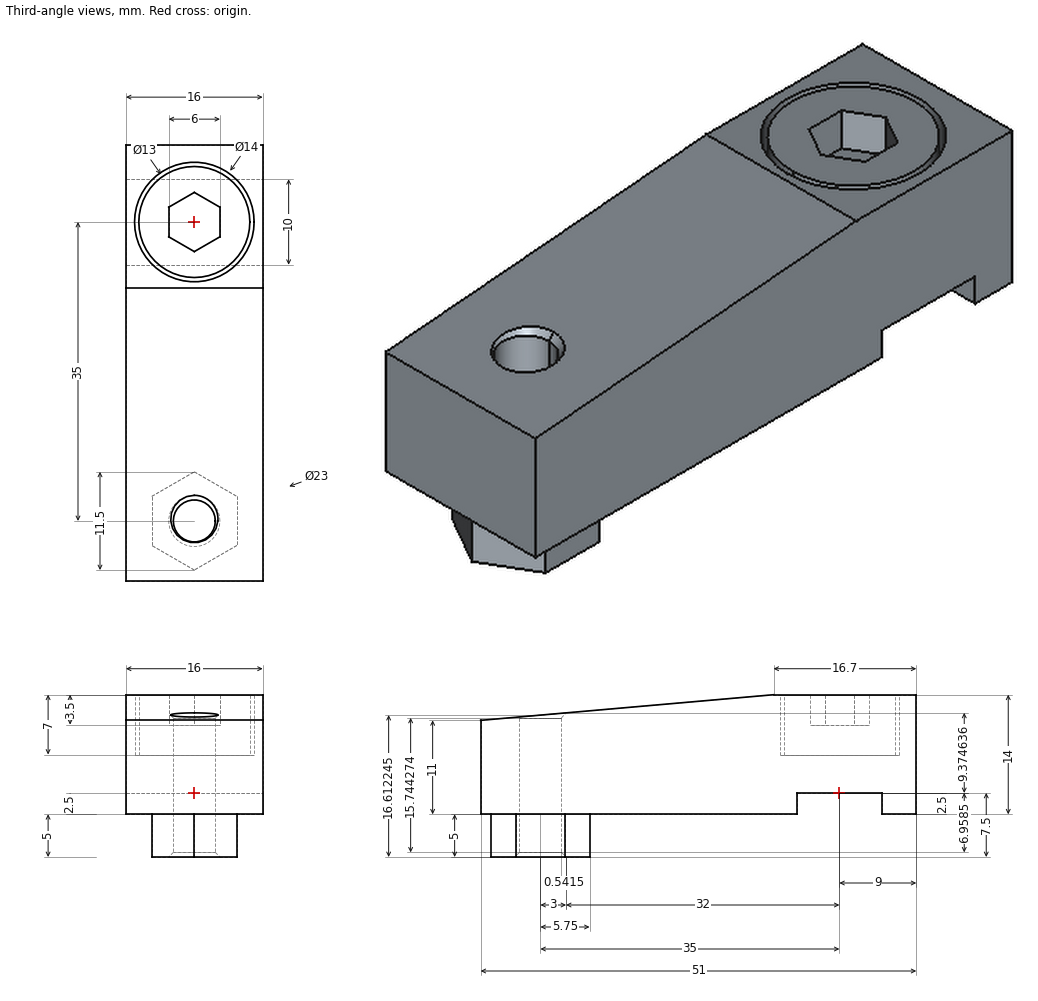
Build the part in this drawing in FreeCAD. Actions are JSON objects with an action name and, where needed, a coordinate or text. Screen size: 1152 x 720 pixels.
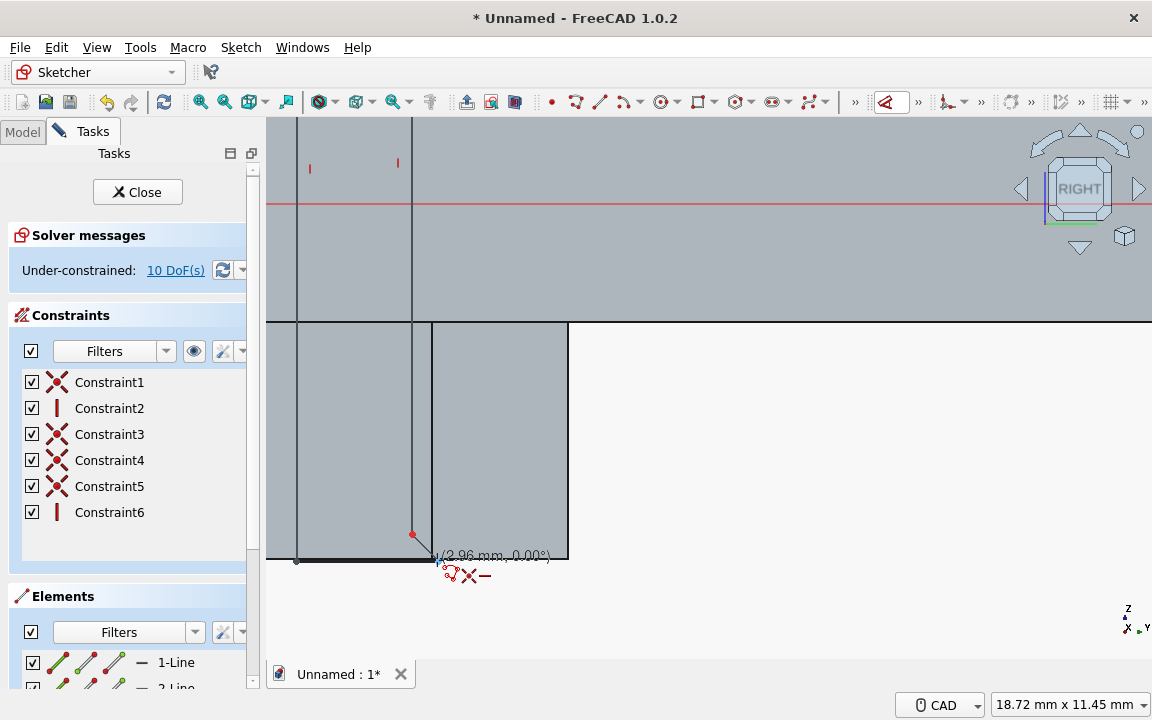
{"action": "left_click", "coordinate": [439, 561]}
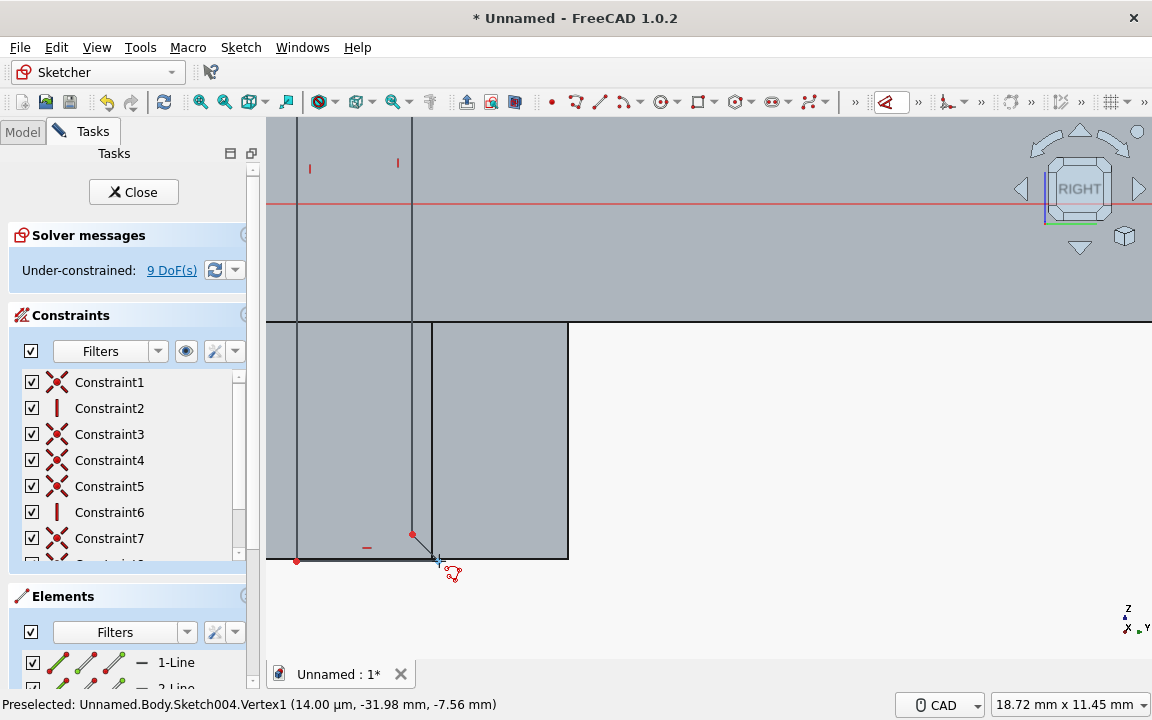
{"action": "left_click", "coordinate": [600, 102]}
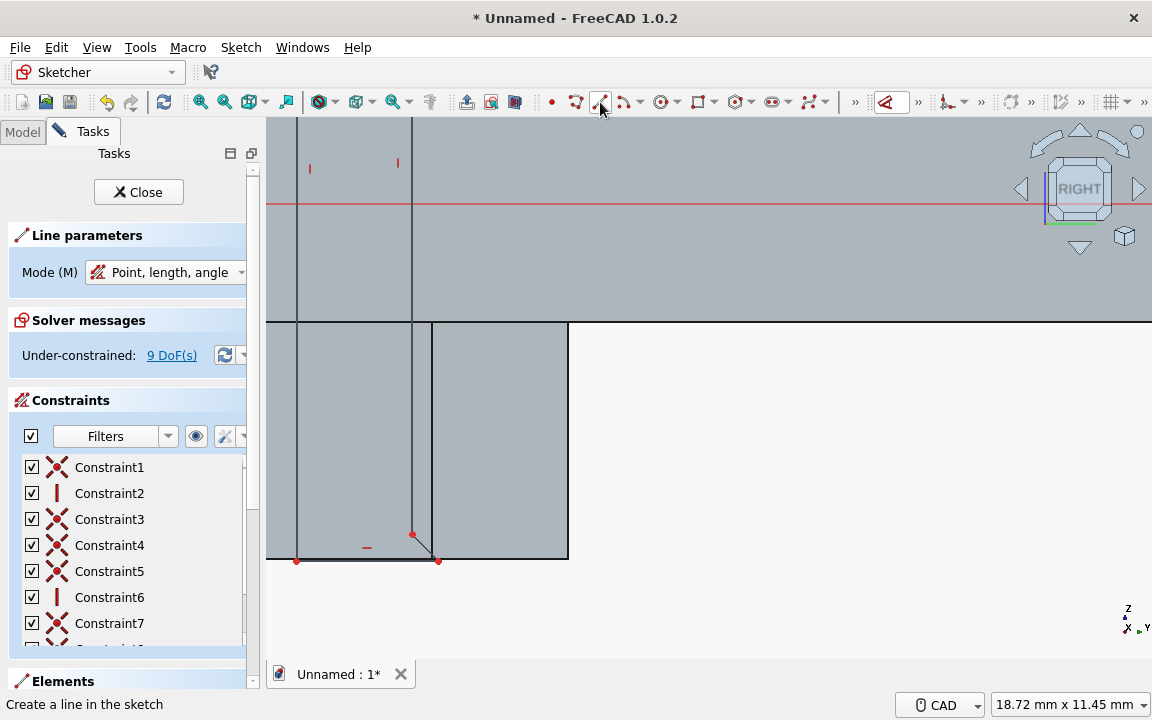
{"action": "scroll", "coordinate": [432, 555], "scroll_direction": "down", "scroll_amount": 6}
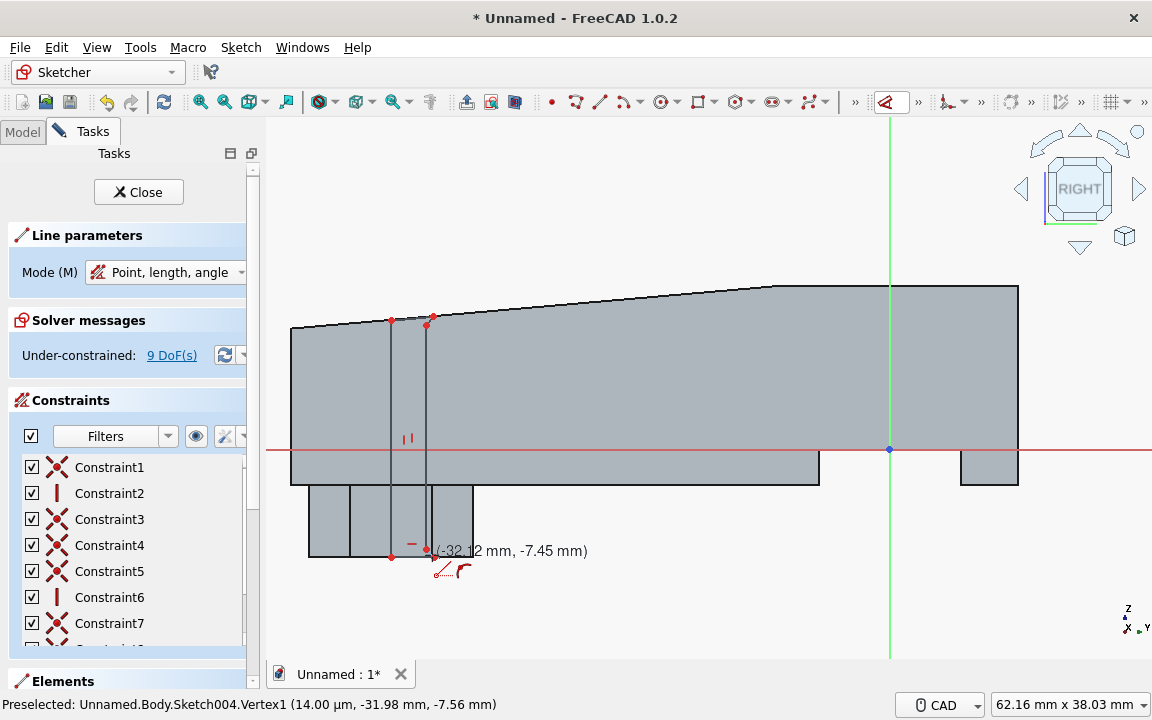
{"action": "left_click", "coordinate": [391, 292]}
{"action": "left_click", "coordinate": [391, 220]}
{"action": "key", "text": "Escape"}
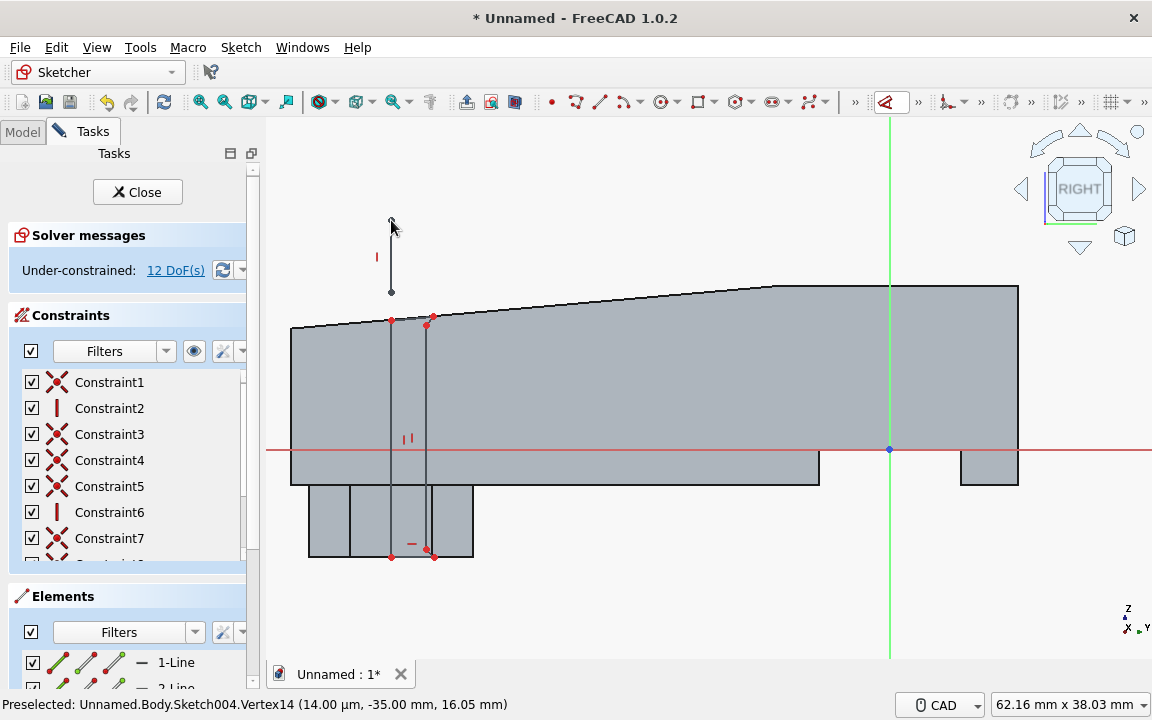
{"action": "left_click", "coordinate": [391, 271]}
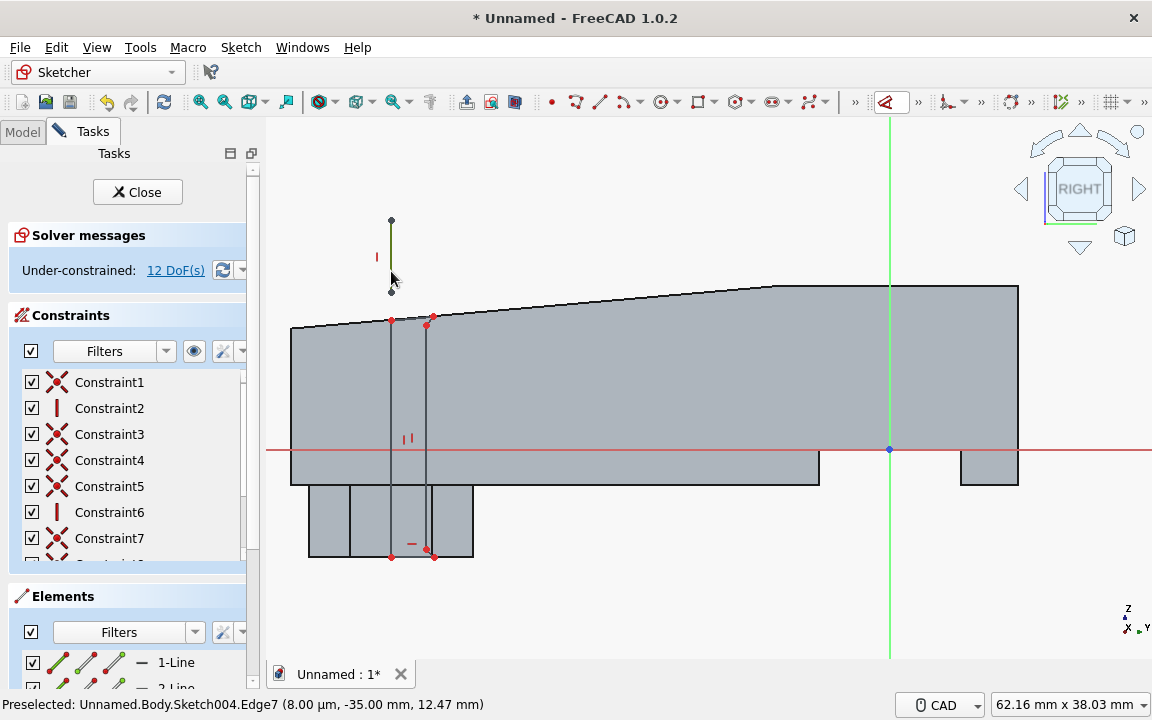
{"action": "key", "text": "g n"}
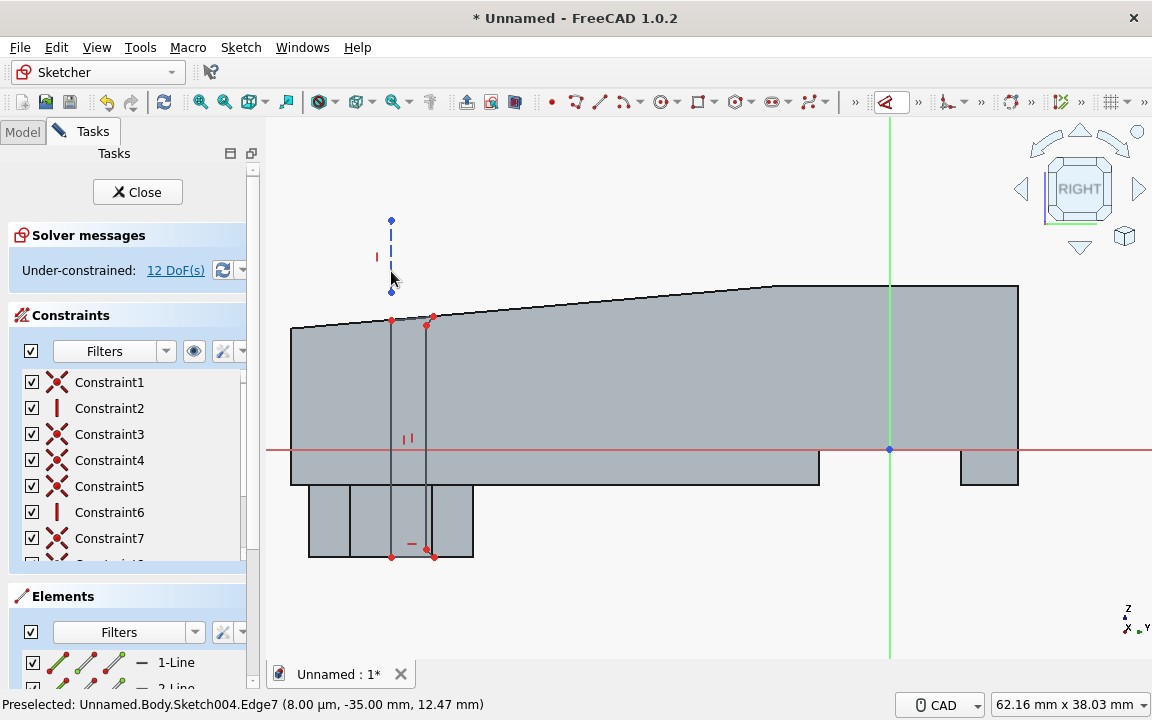
{"action": "left_click", "coordinate": [404, 557]}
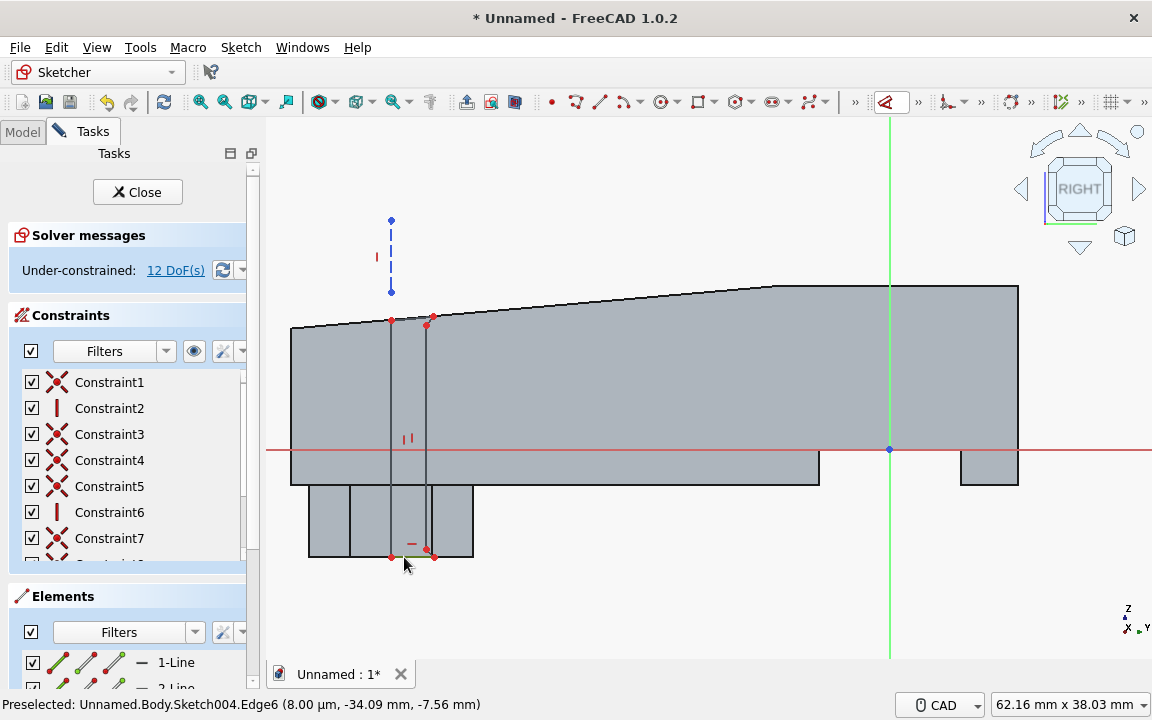
{"action": "key", "text": "l"}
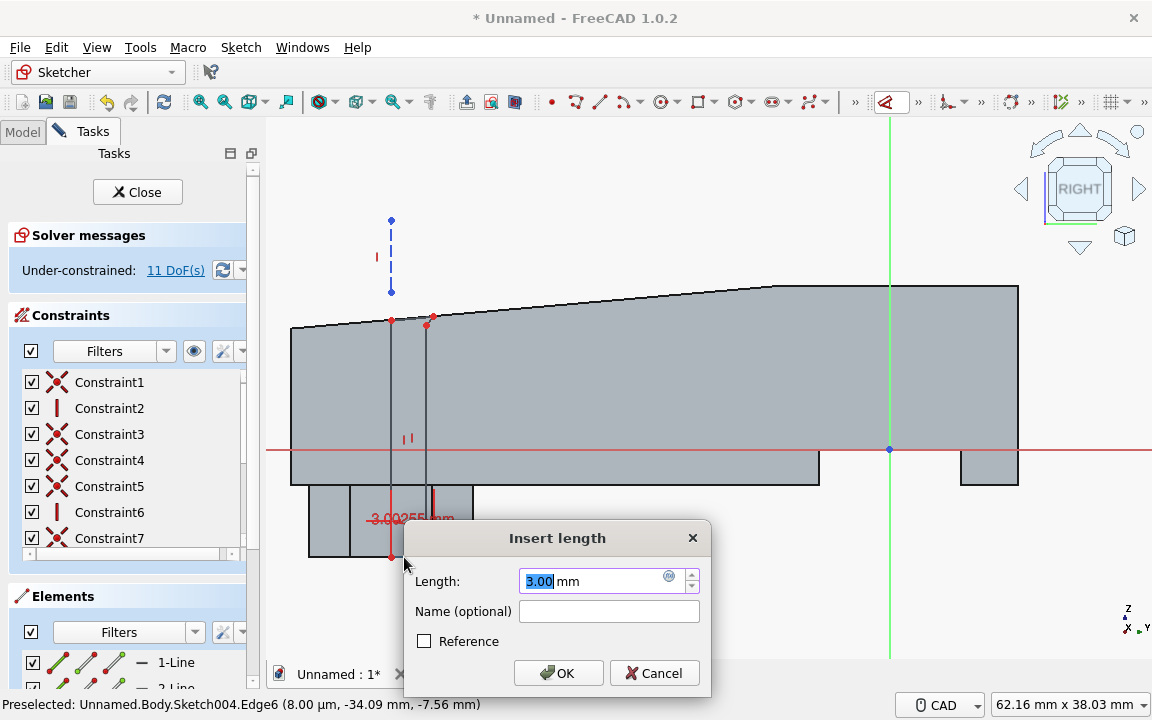
{"action": "type", "text": "3"}
{"action": "key", "text": "Return"}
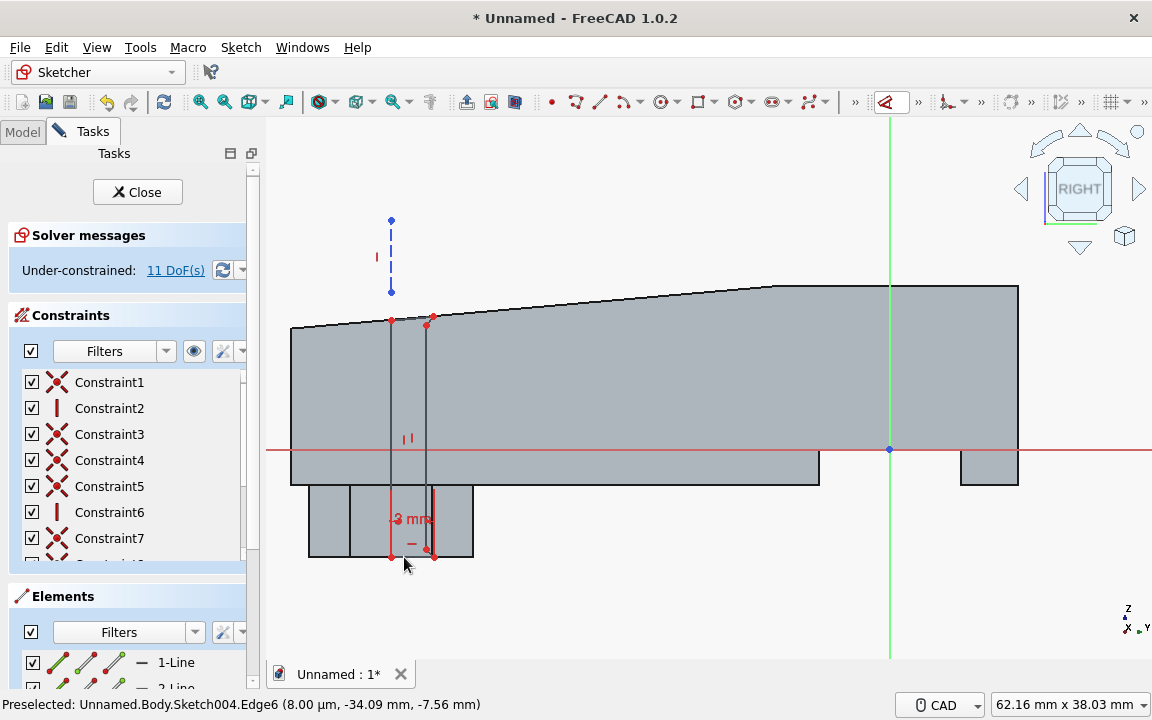
{"action": "left_click", "coordinate": [404, 320]}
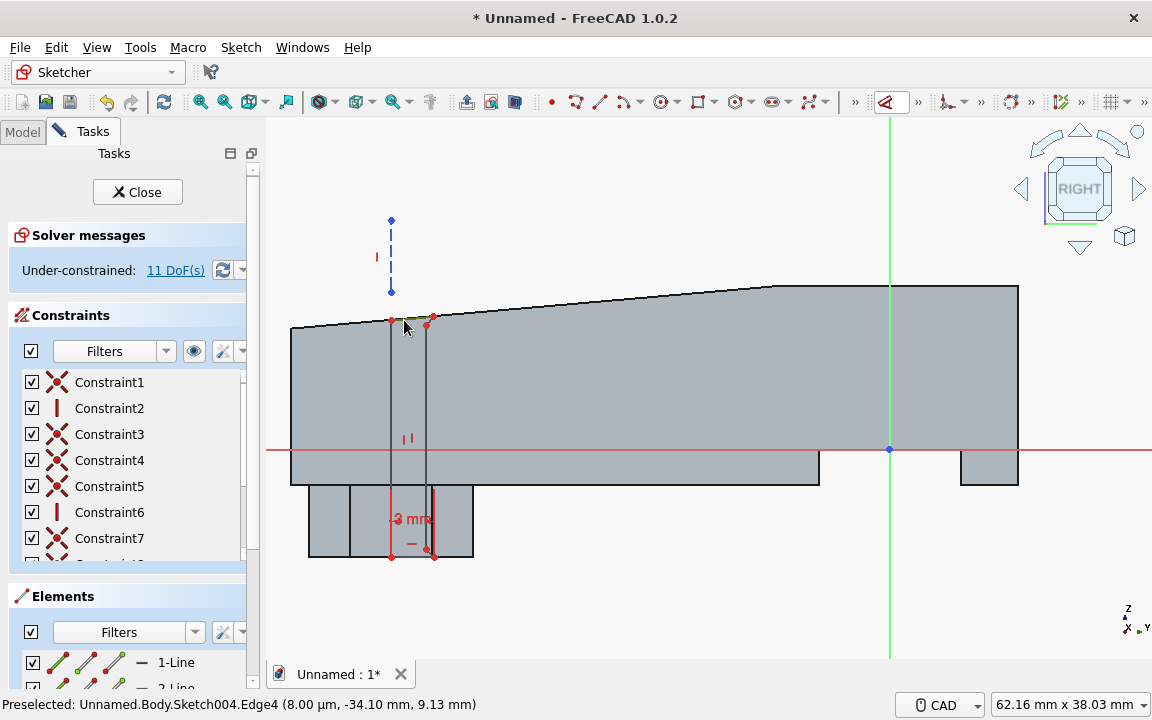
{"action": "left_click", "coordinate": [904, 102]}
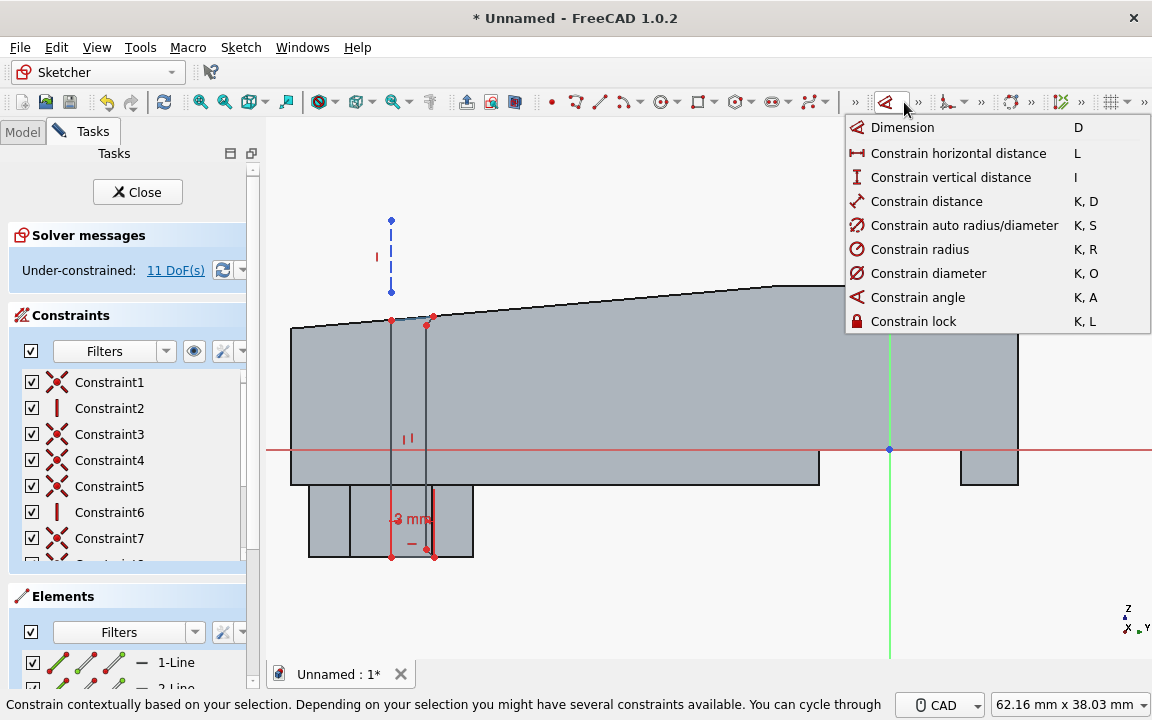
{"action": "left_click", "coordinate": [998, 153]}